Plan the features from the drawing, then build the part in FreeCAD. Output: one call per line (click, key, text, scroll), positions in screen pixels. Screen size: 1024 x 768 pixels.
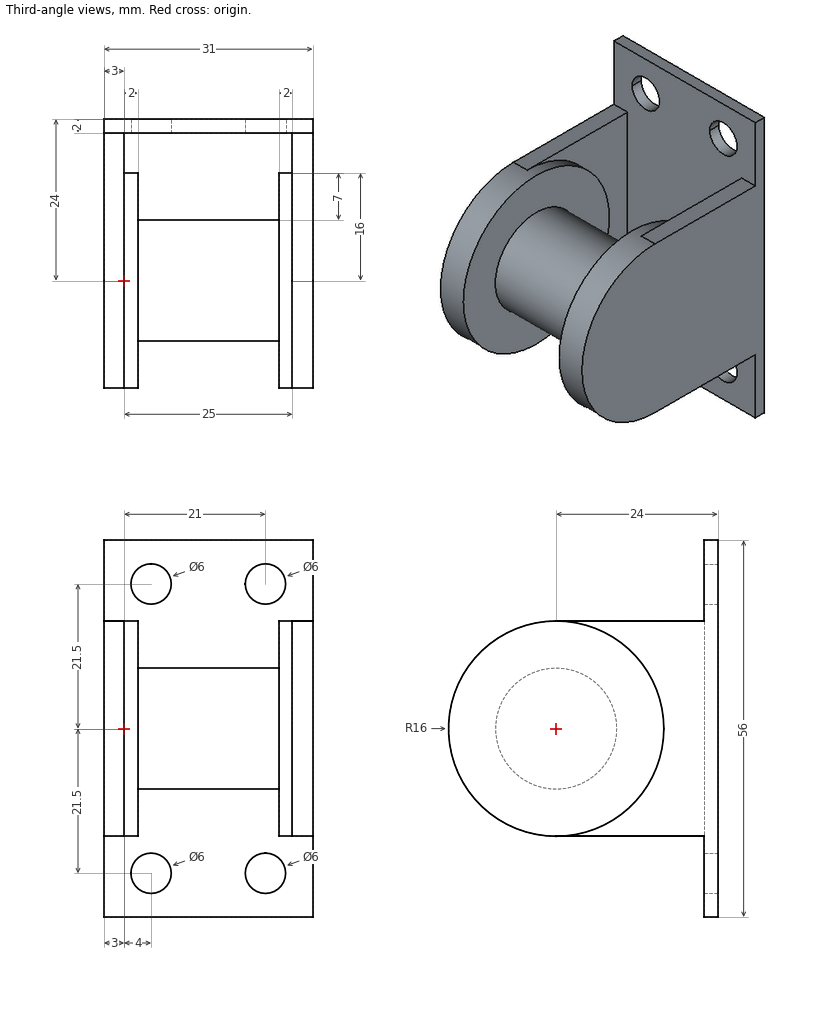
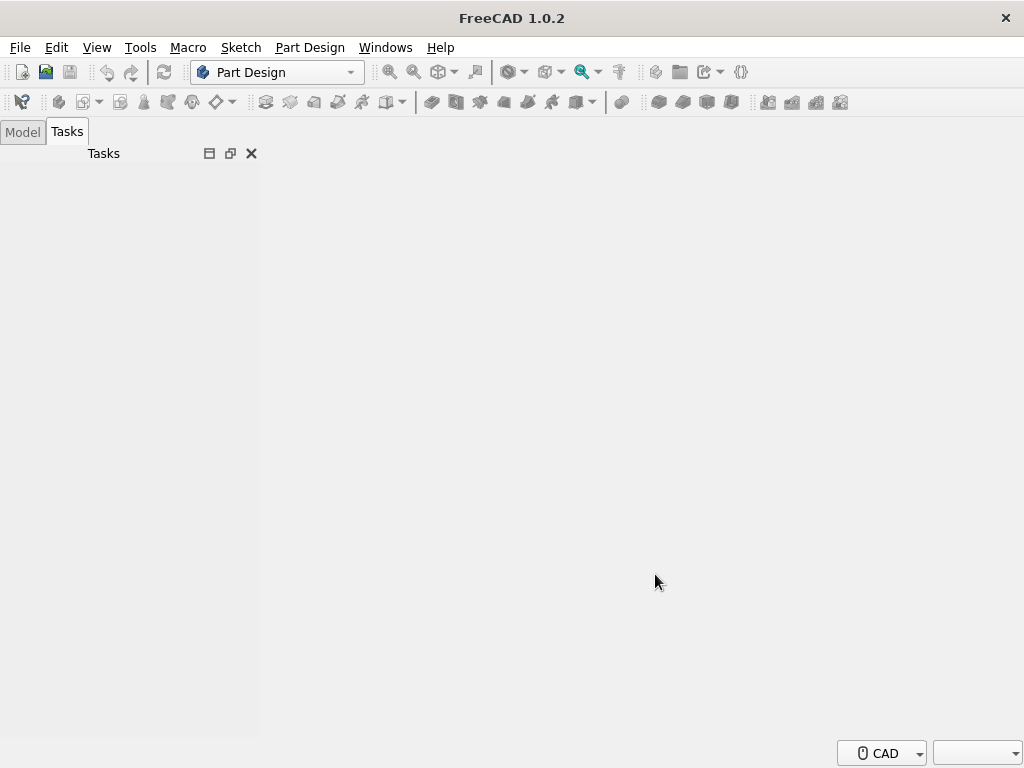
click(22, 72)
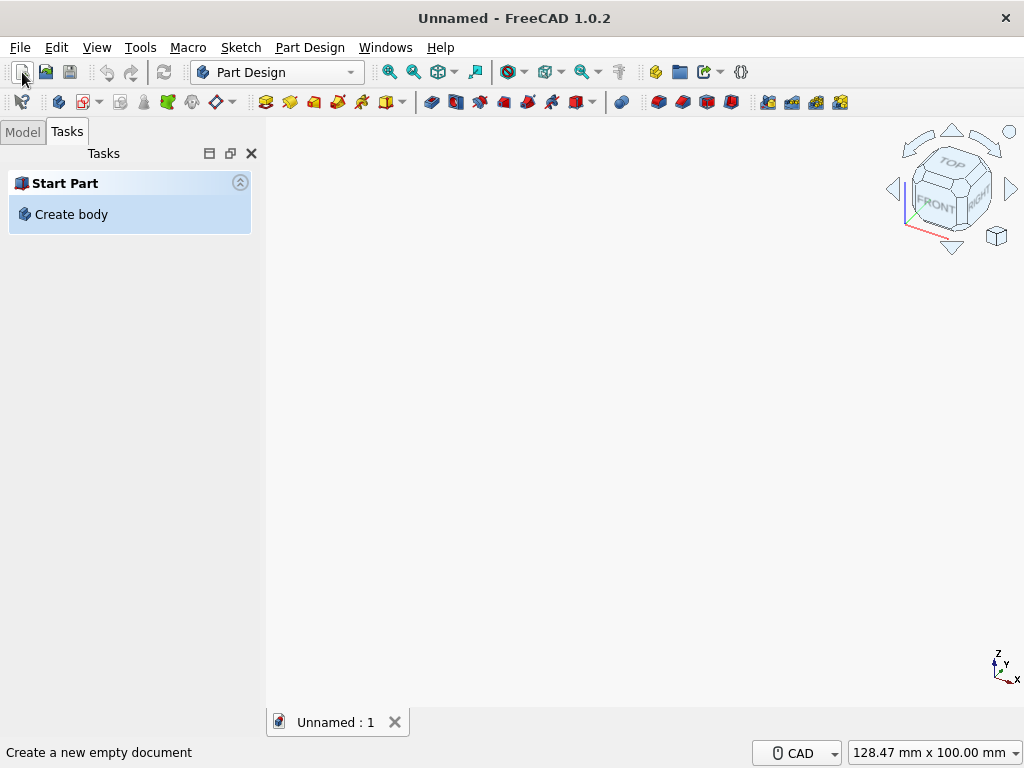
click(84, 102)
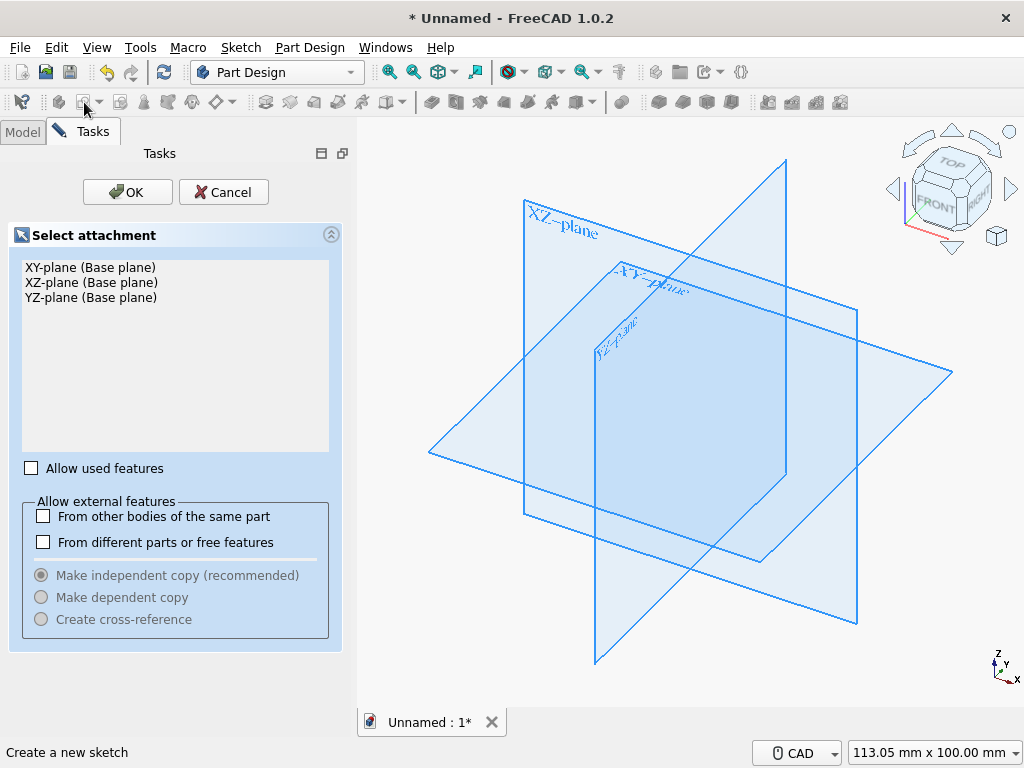
click(82, 268)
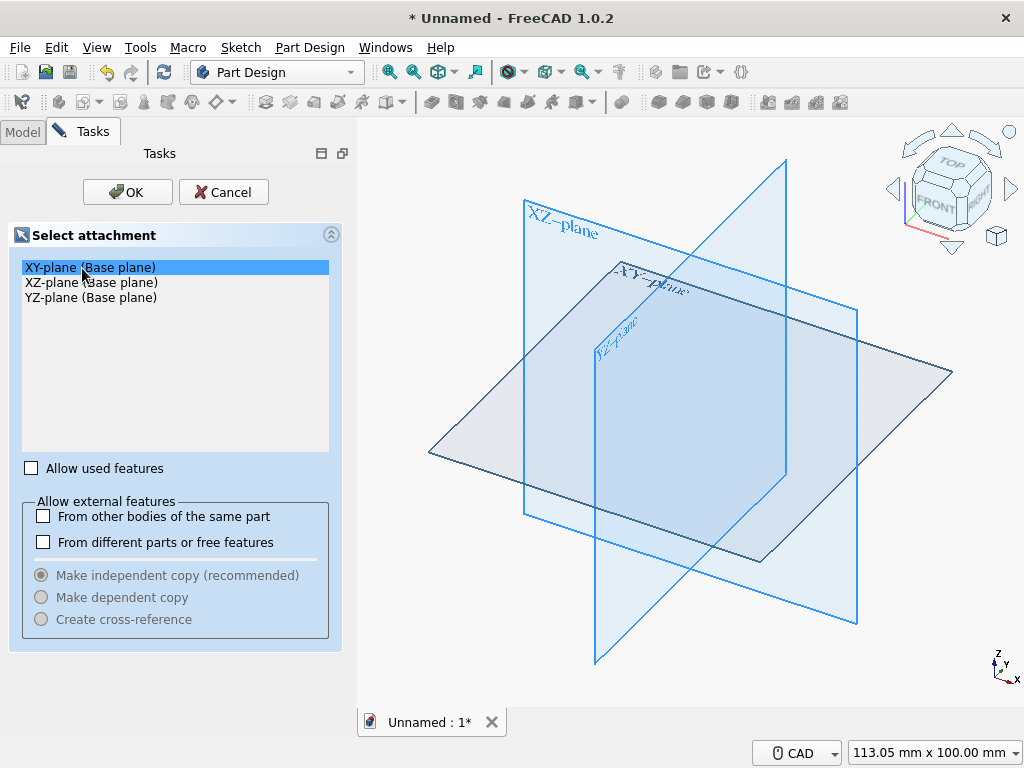
click(128, 192)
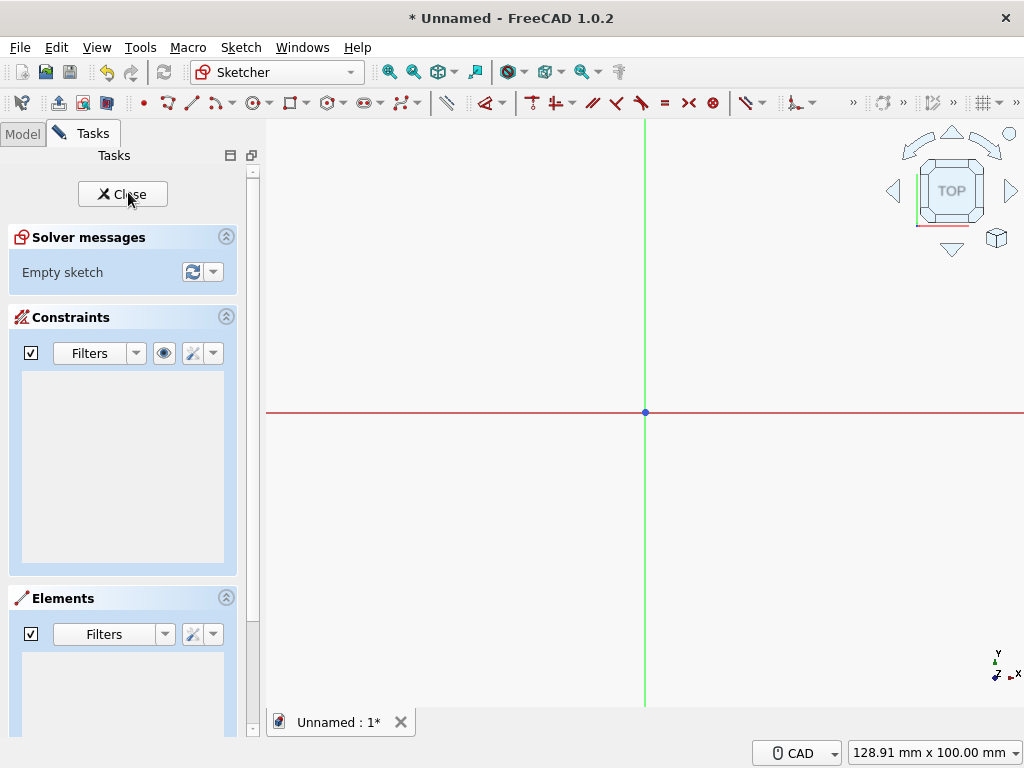
scroll(801, 339, up, 5)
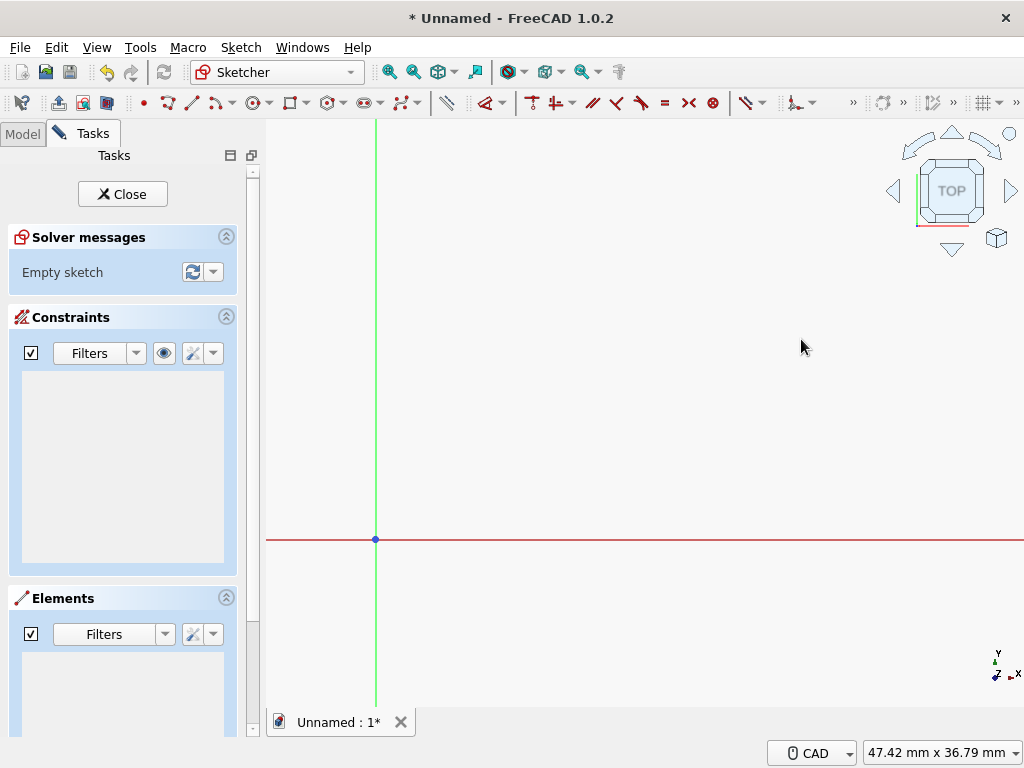
click(168, 104)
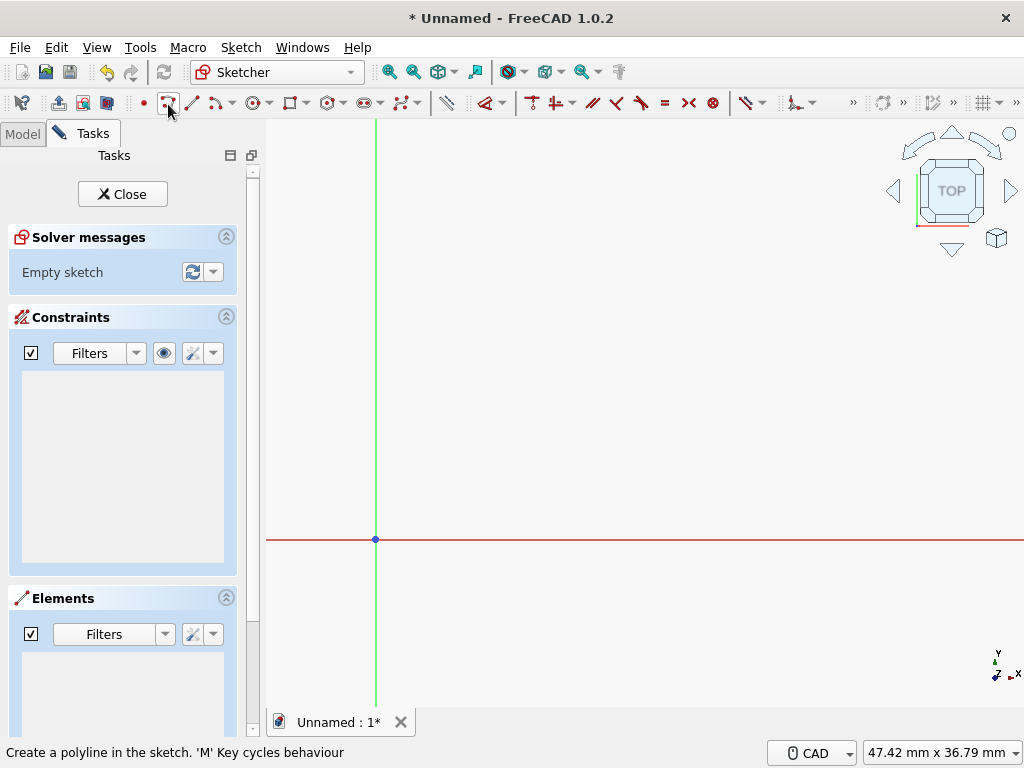
click(376, 540)
click(775, 531)
click(775, 284)
click(743, 284)
click(743, 396)
click(408, 396)
click(408, 284)
click(385, 284)
click(376, 540)
key(Escape)
key(Escape)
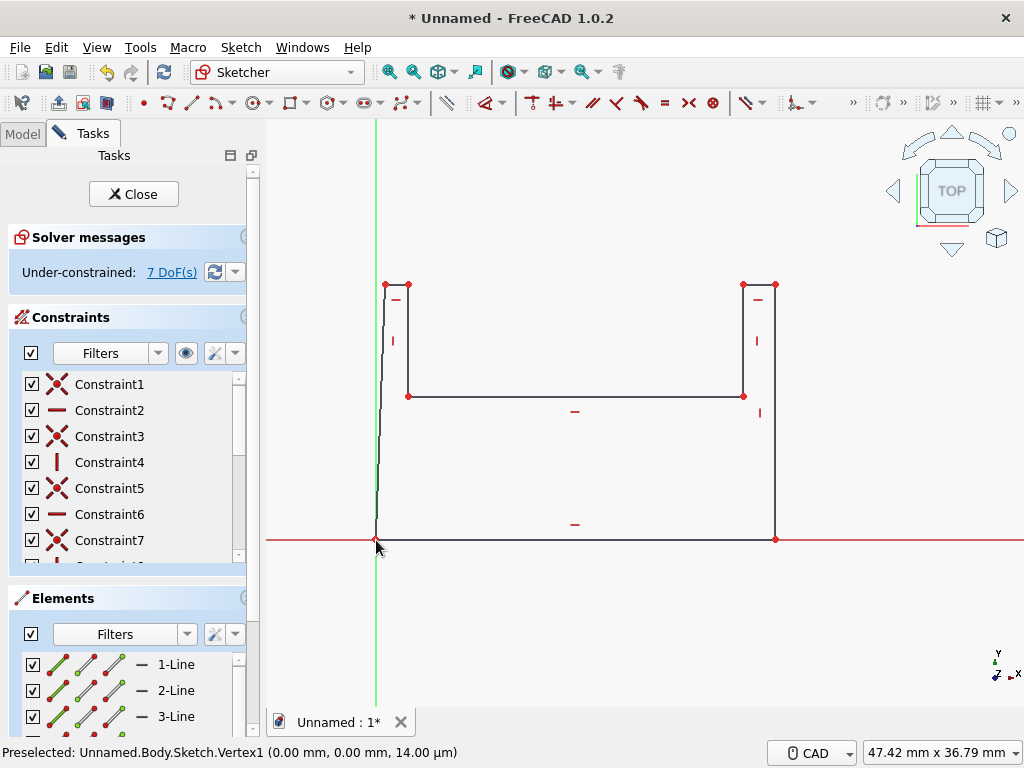
click(379, 463)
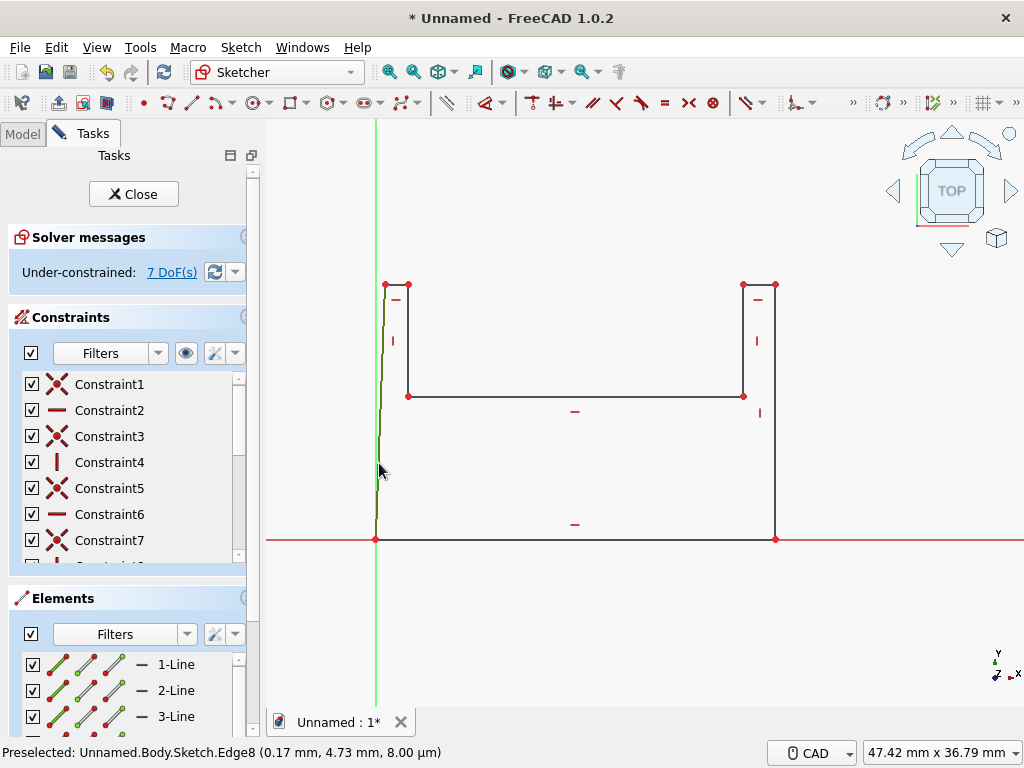
key(v)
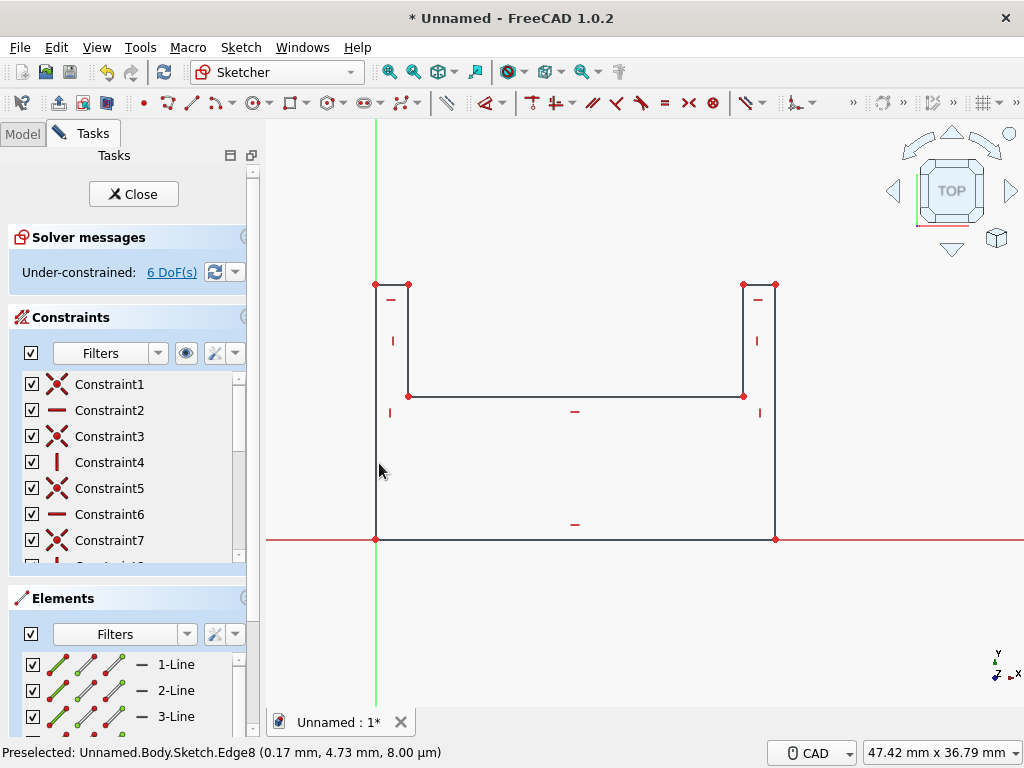
click(486, 104)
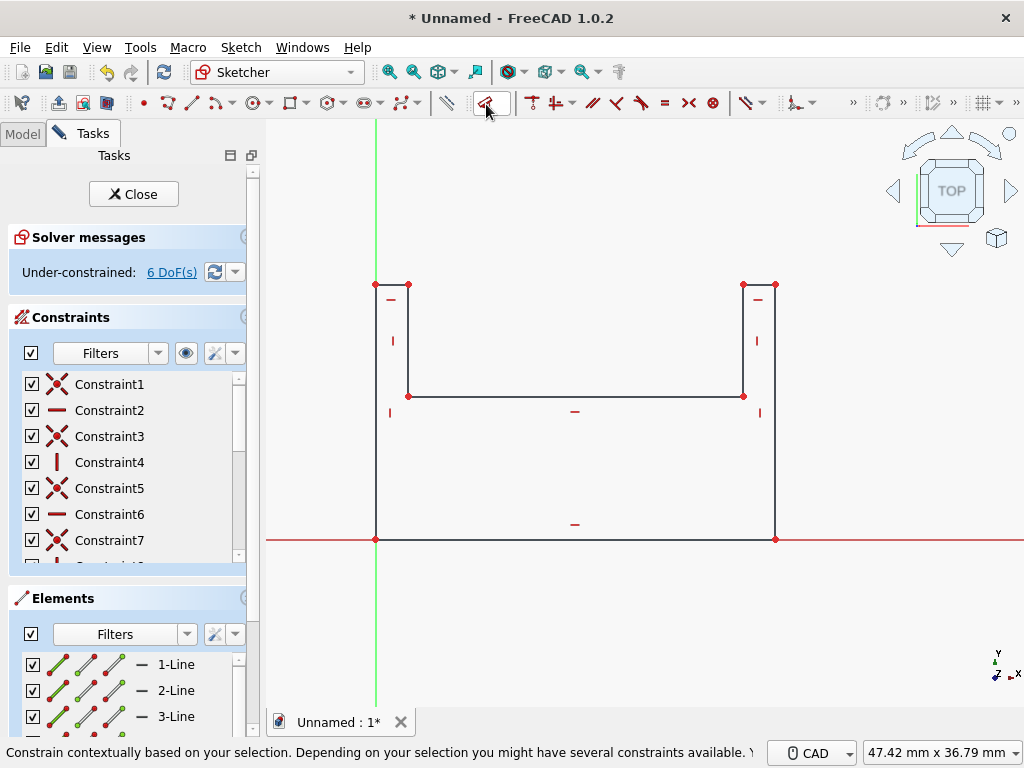
scroll(765, 285, up, 2)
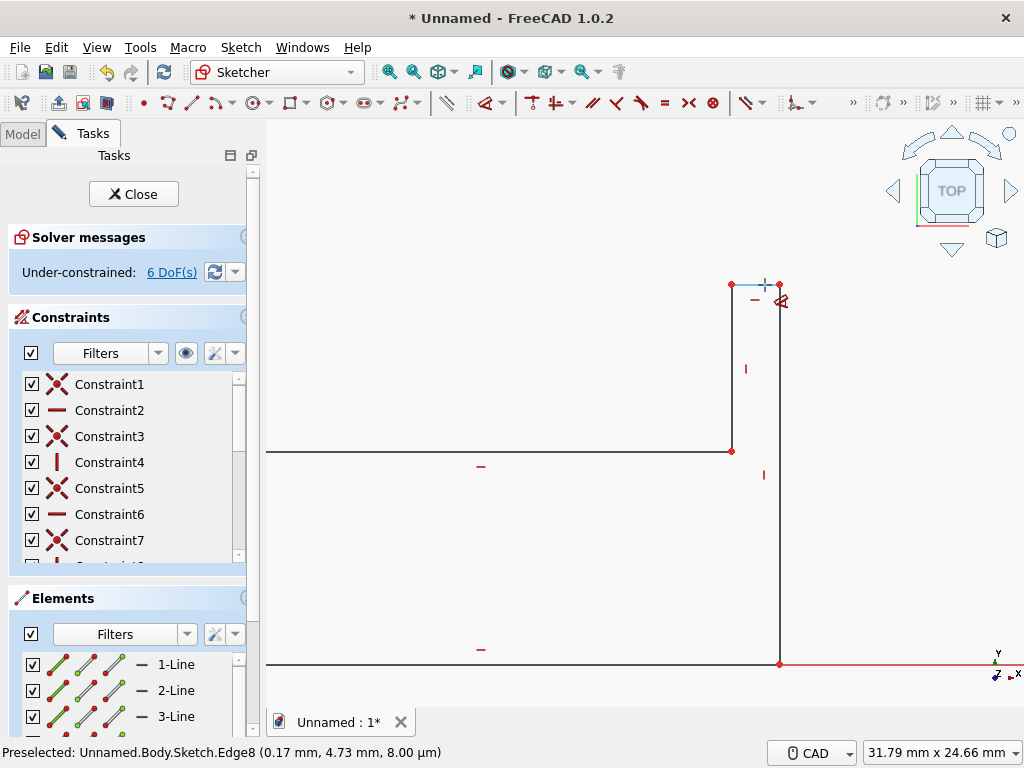
click(765, 285)
click(756, 251)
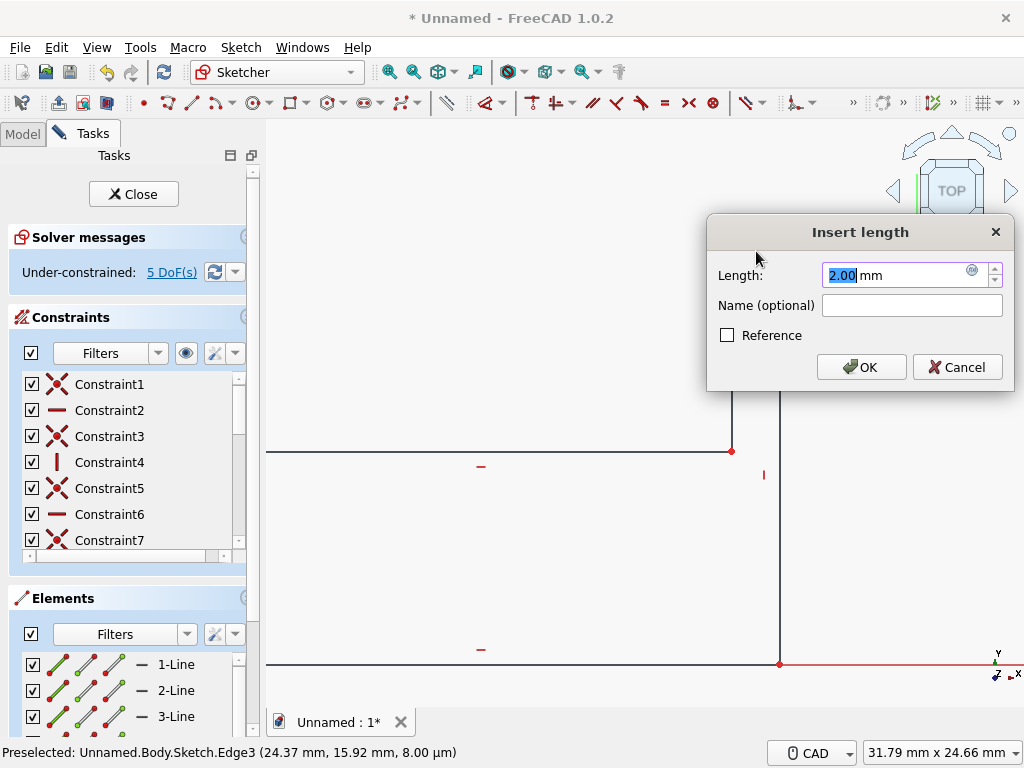
text(2)
key(Return)